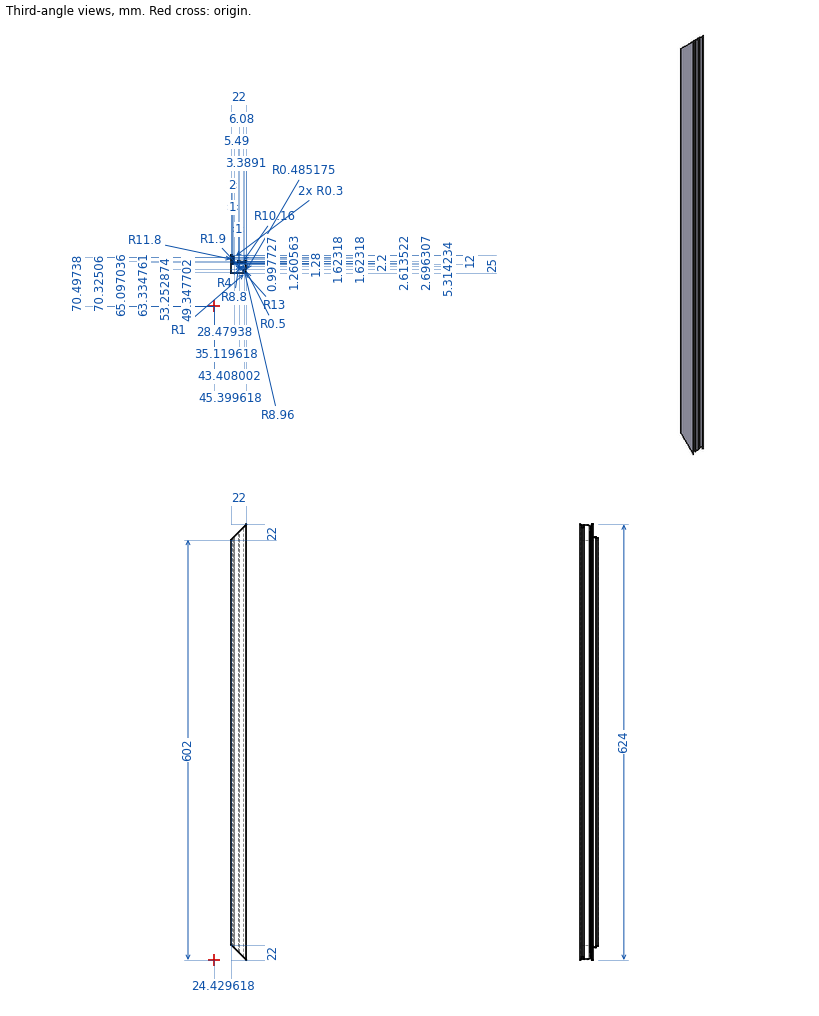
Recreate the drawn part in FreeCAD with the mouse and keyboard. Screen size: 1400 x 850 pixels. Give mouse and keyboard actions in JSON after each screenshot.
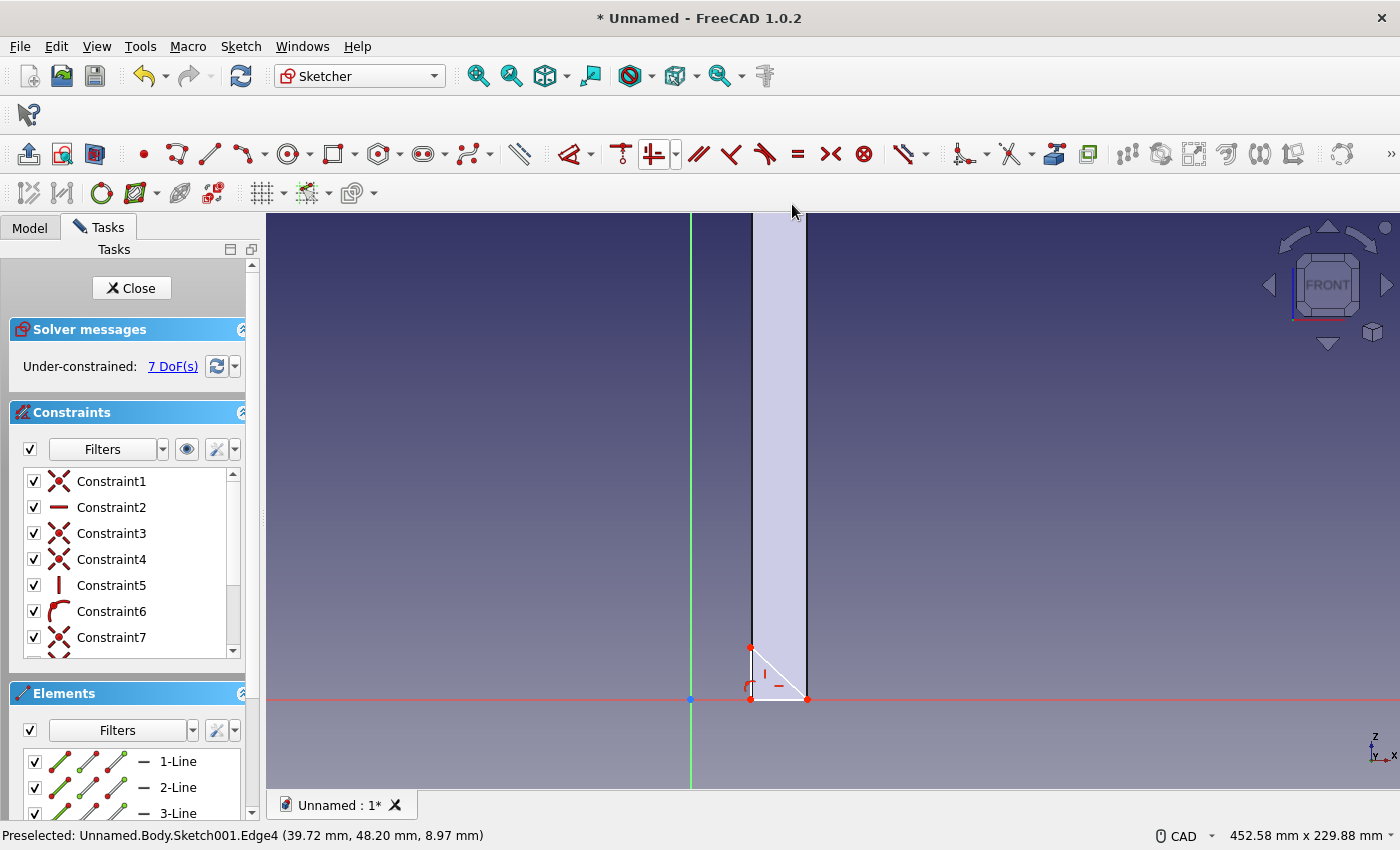
{"action": "left_click", "coordinate": [568, 154]}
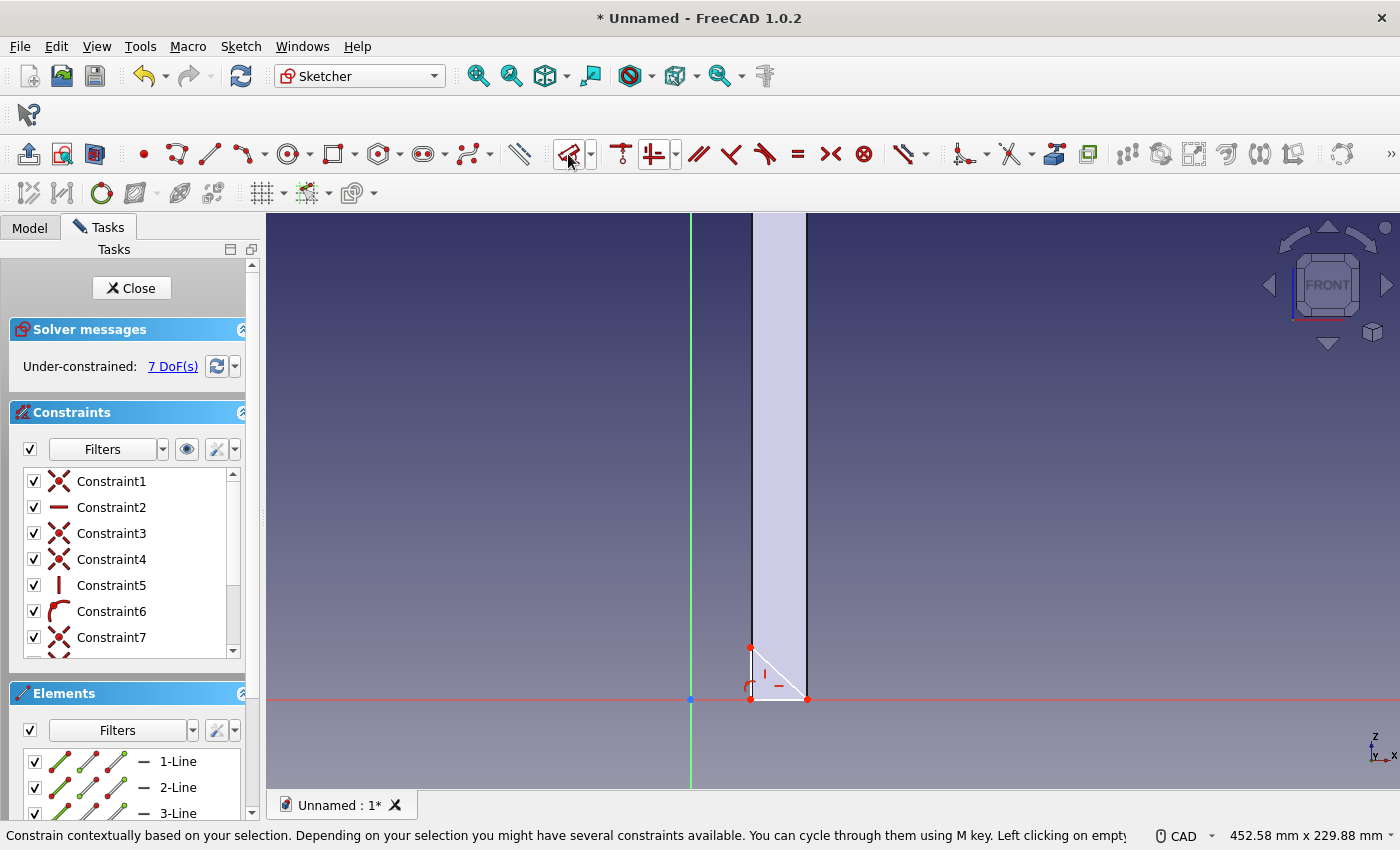
{"action": "scroll", "coordinate": [770, 692], "scroll_direction": "down", "scroll_amount": 7}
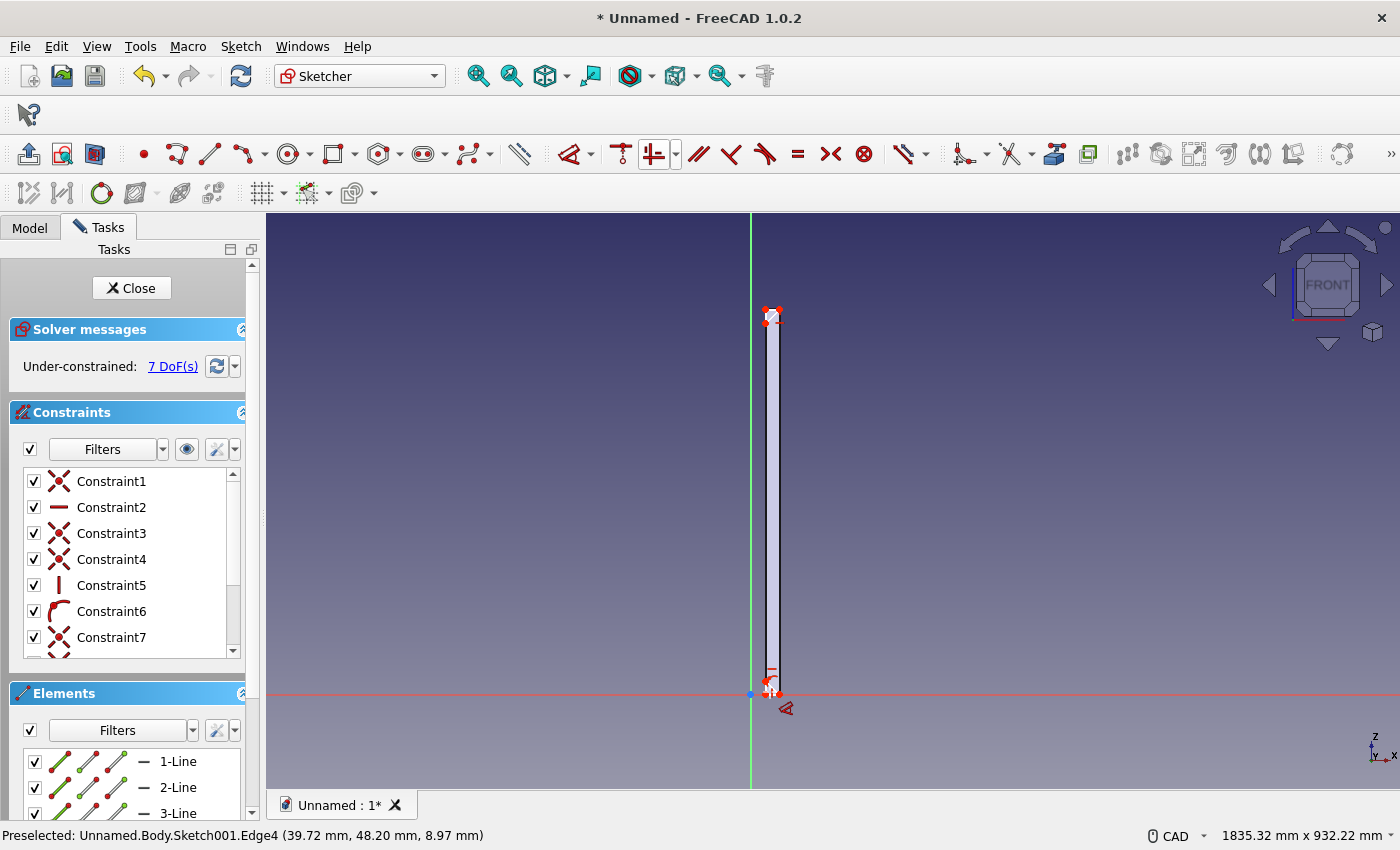
{"action": "scroll", "coordinate": [775, 310], "scroll_direction": "up", "scroll_amount": 8}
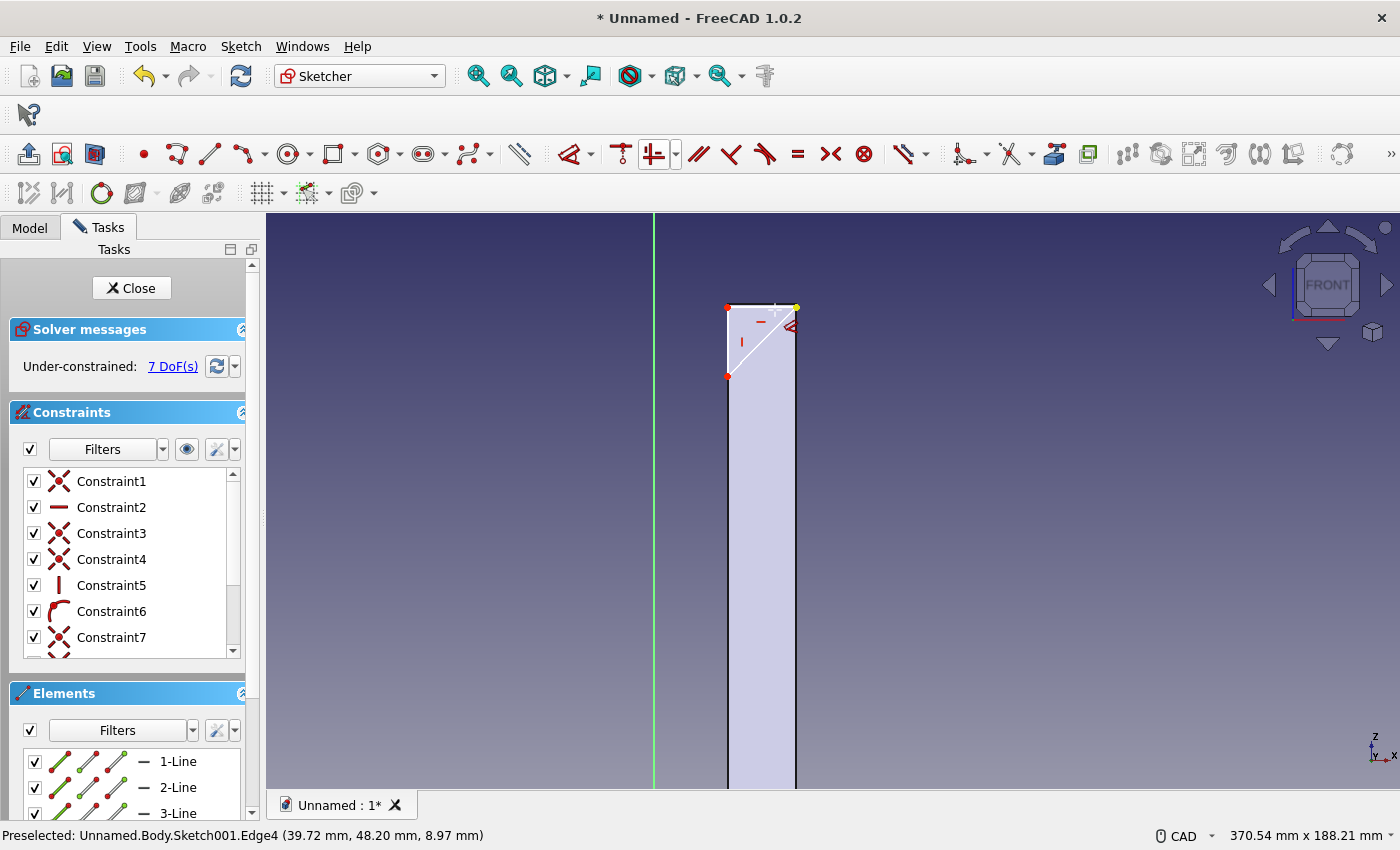
{"action": "left_click", "coordinate": [776, 307]}
{"action": "left_click", "coordinate": [762, 273]}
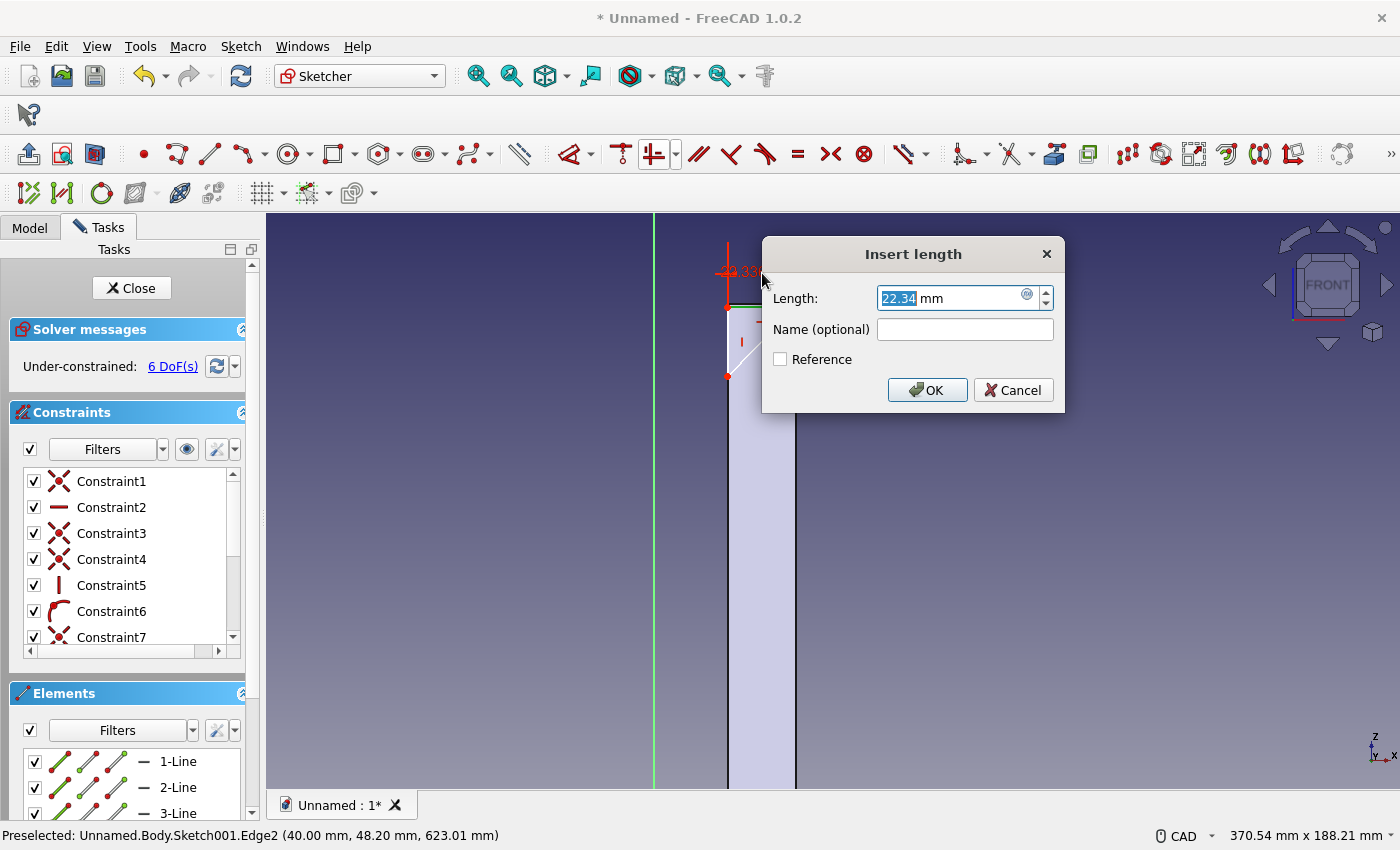
{"action": "type", "text": "22"}
{"action": "key", "text": "Return"}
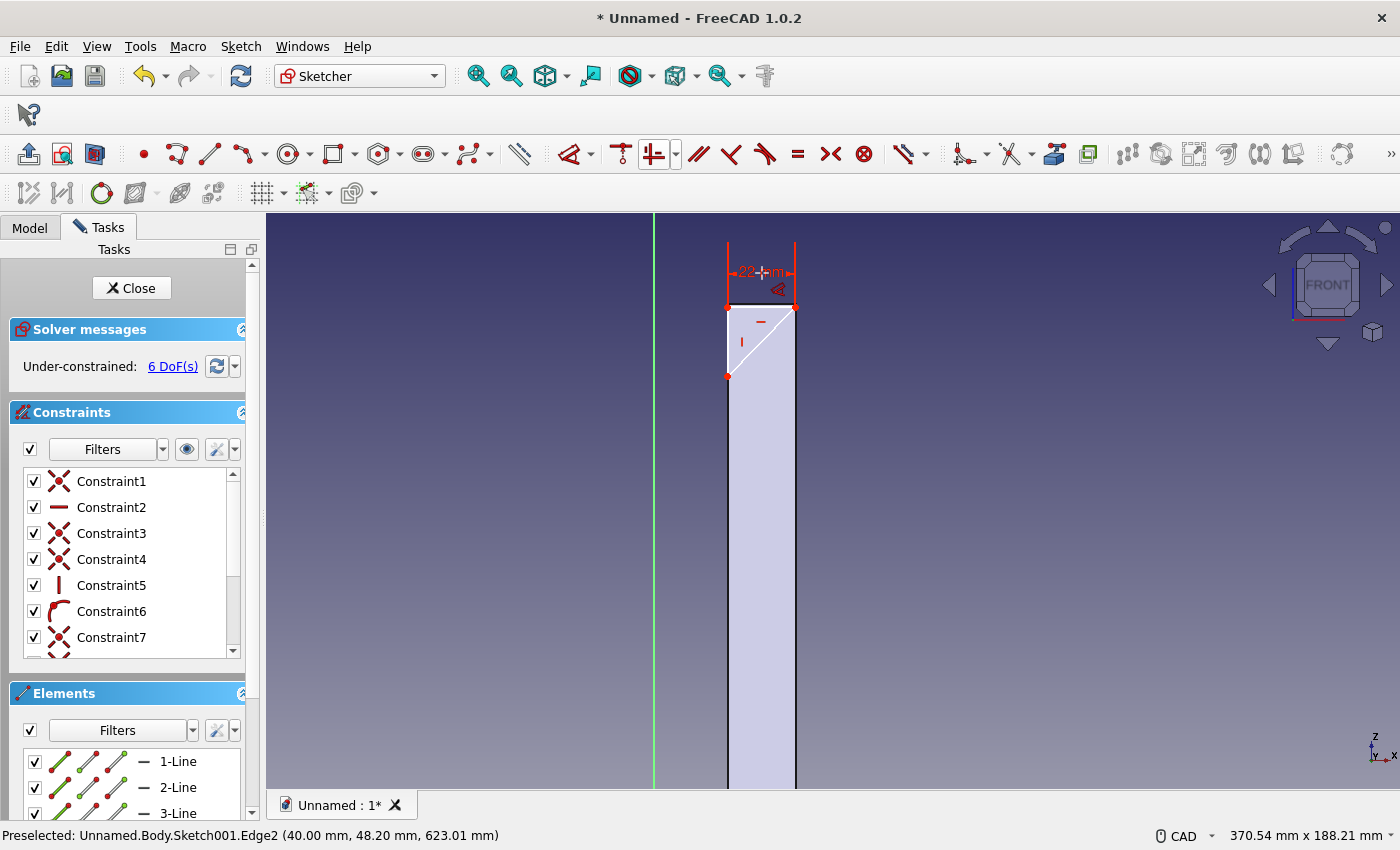
{"action": "left_click", "coordinate": [728, 328]}
{"action": "left_click", "coordinate": [762, 366]}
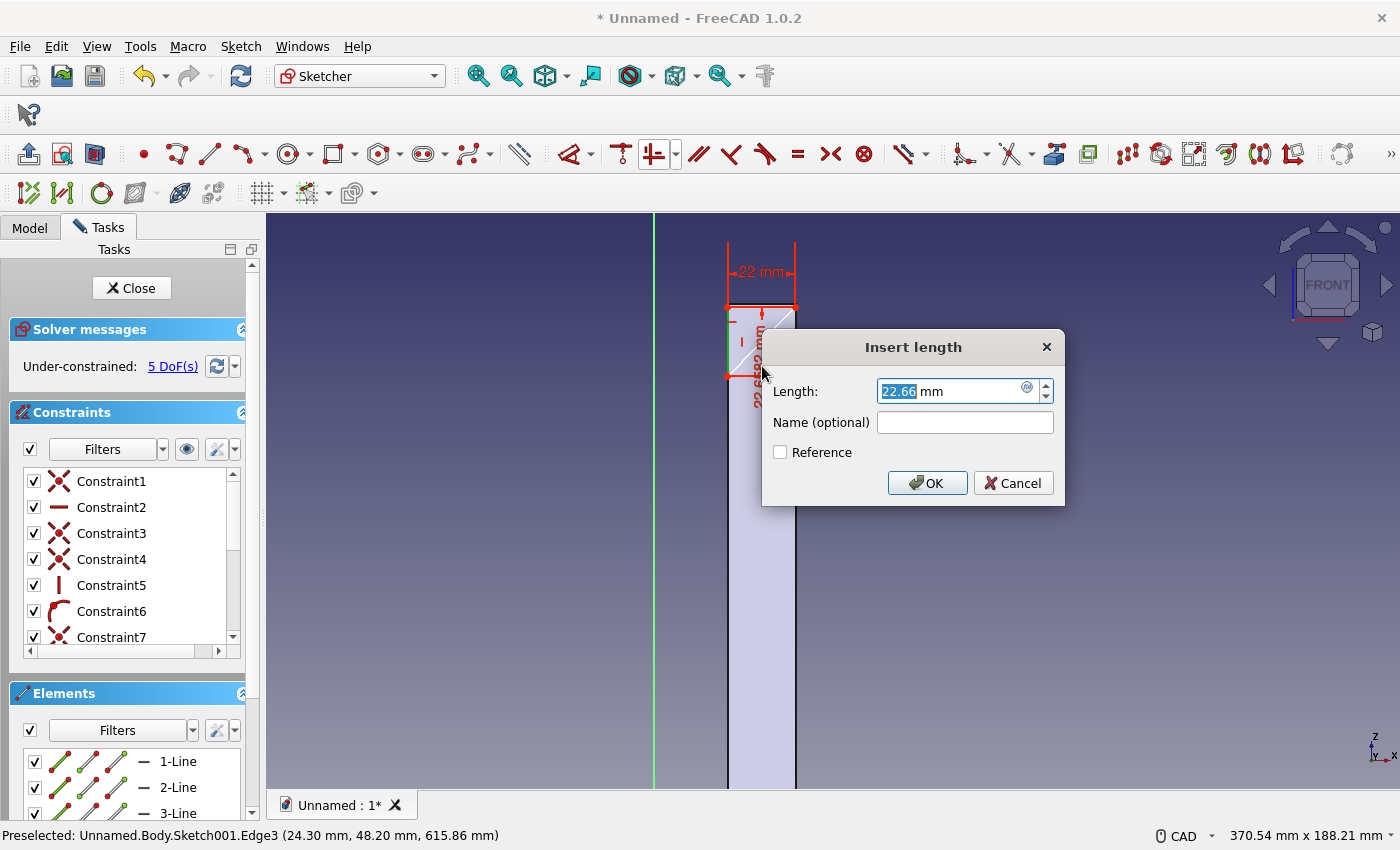
{"action": "type", "text": "22"}
{"action": "key", "text": "Return"}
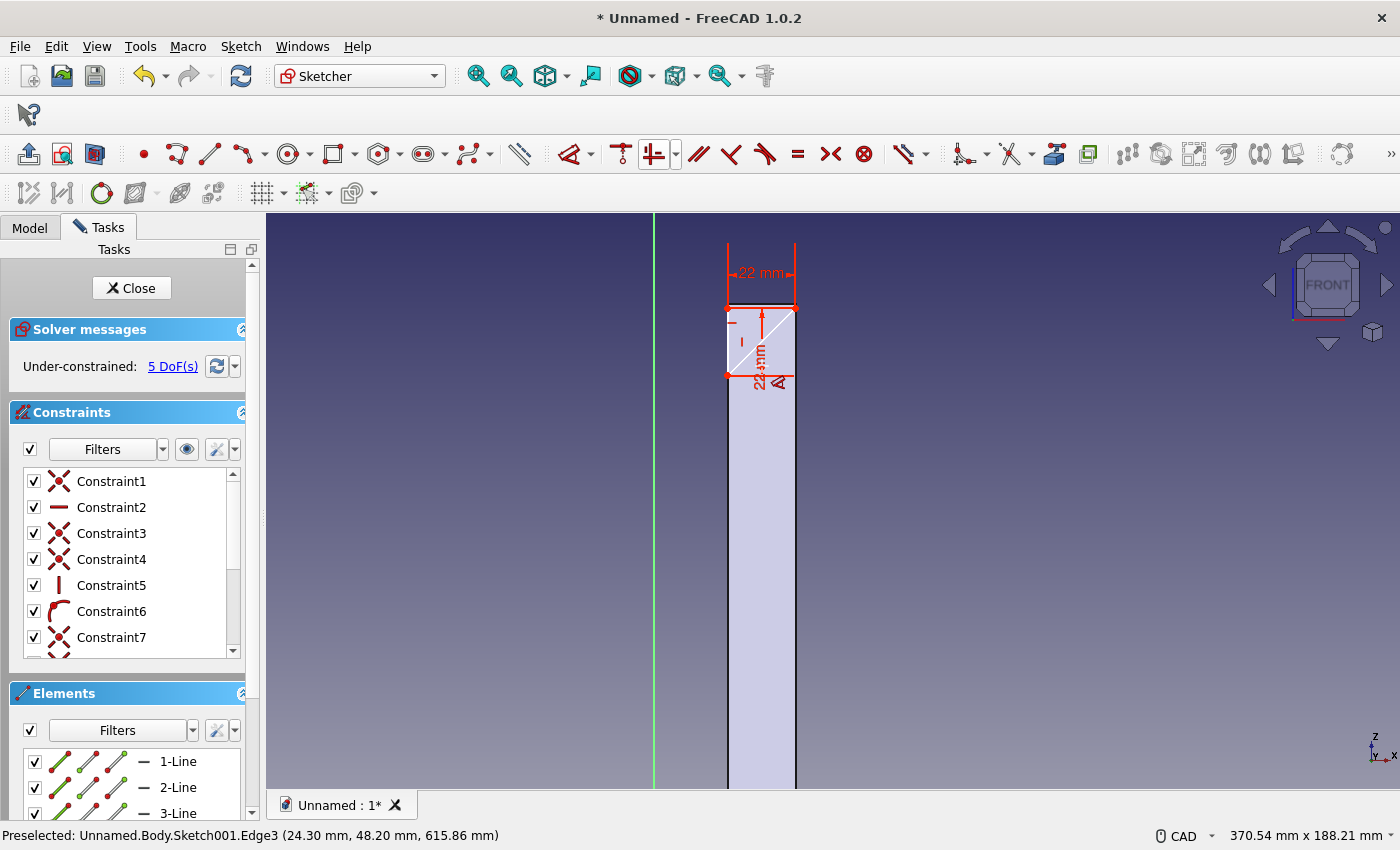
{"action": "scroll", "coordinate": [775, 309], "scroll_direction": "down", "scroll_amount": 8}